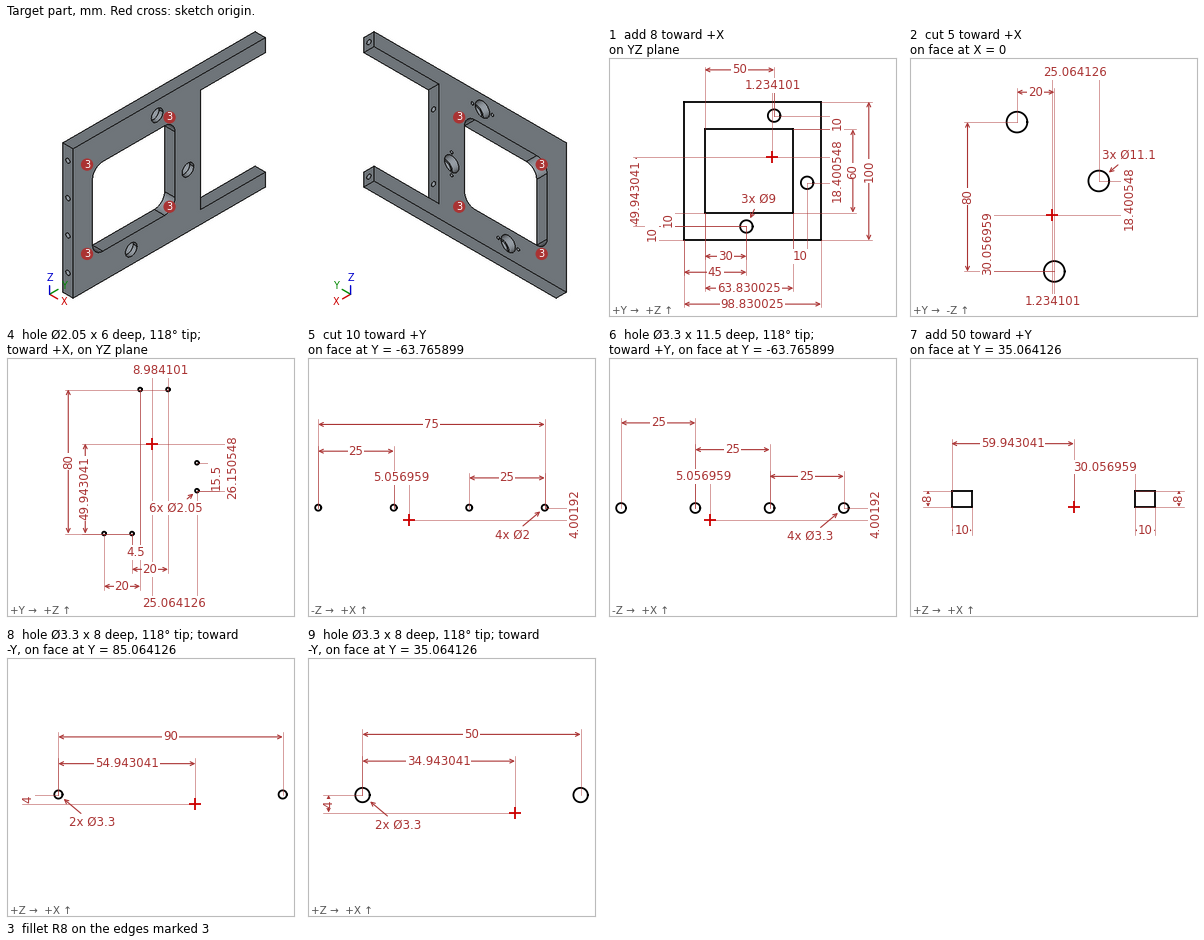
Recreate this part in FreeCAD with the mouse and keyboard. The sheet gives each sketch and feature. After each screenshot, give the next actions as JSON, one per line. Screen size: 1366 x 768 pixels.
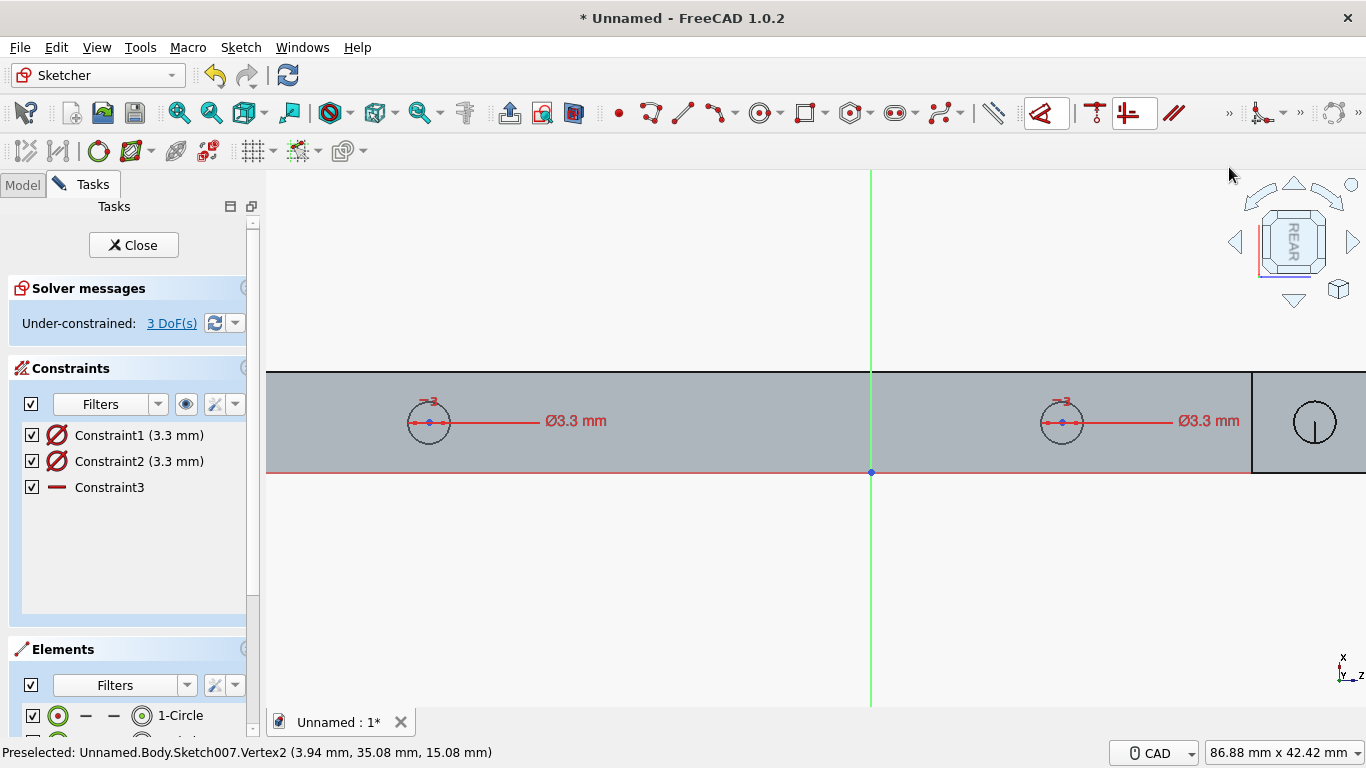
{"action": "left_click", "coordinate": [429, 423]}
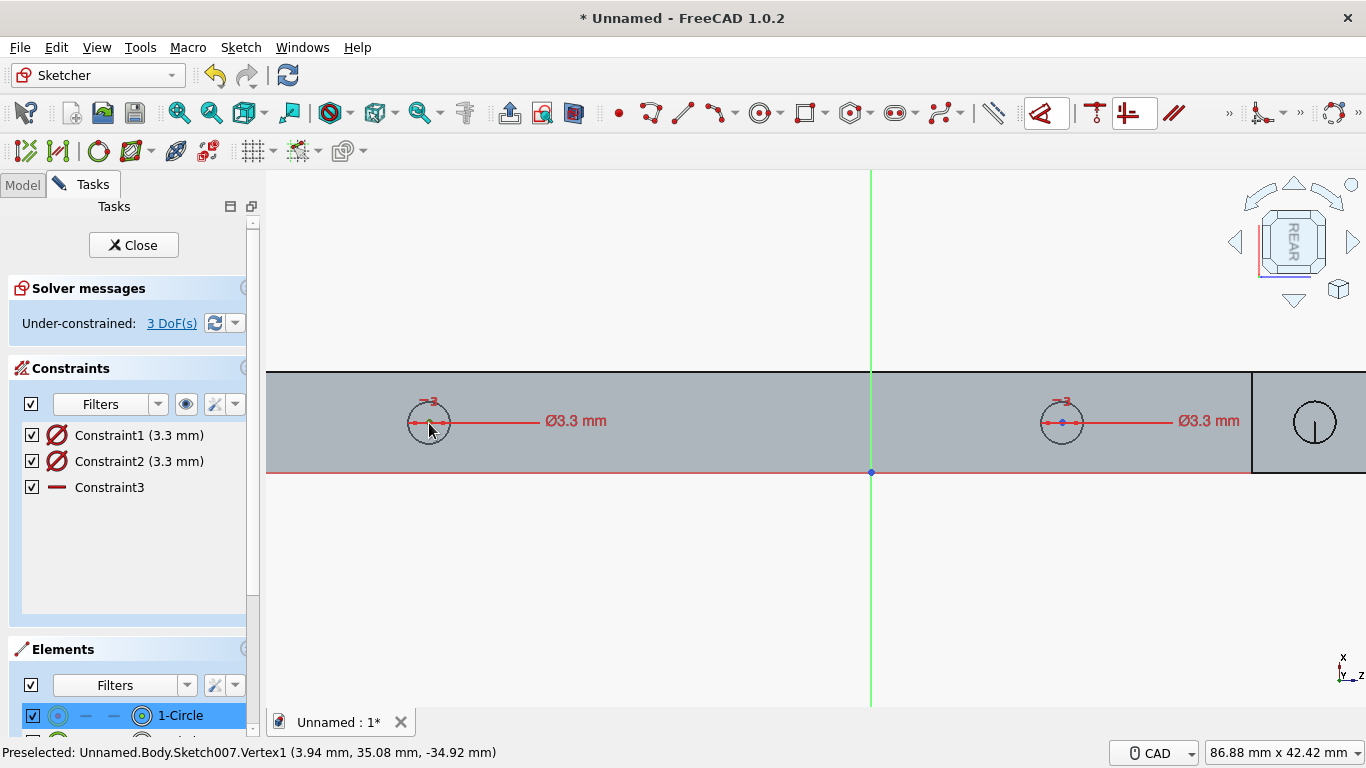
{"action": "key", "text": "i"}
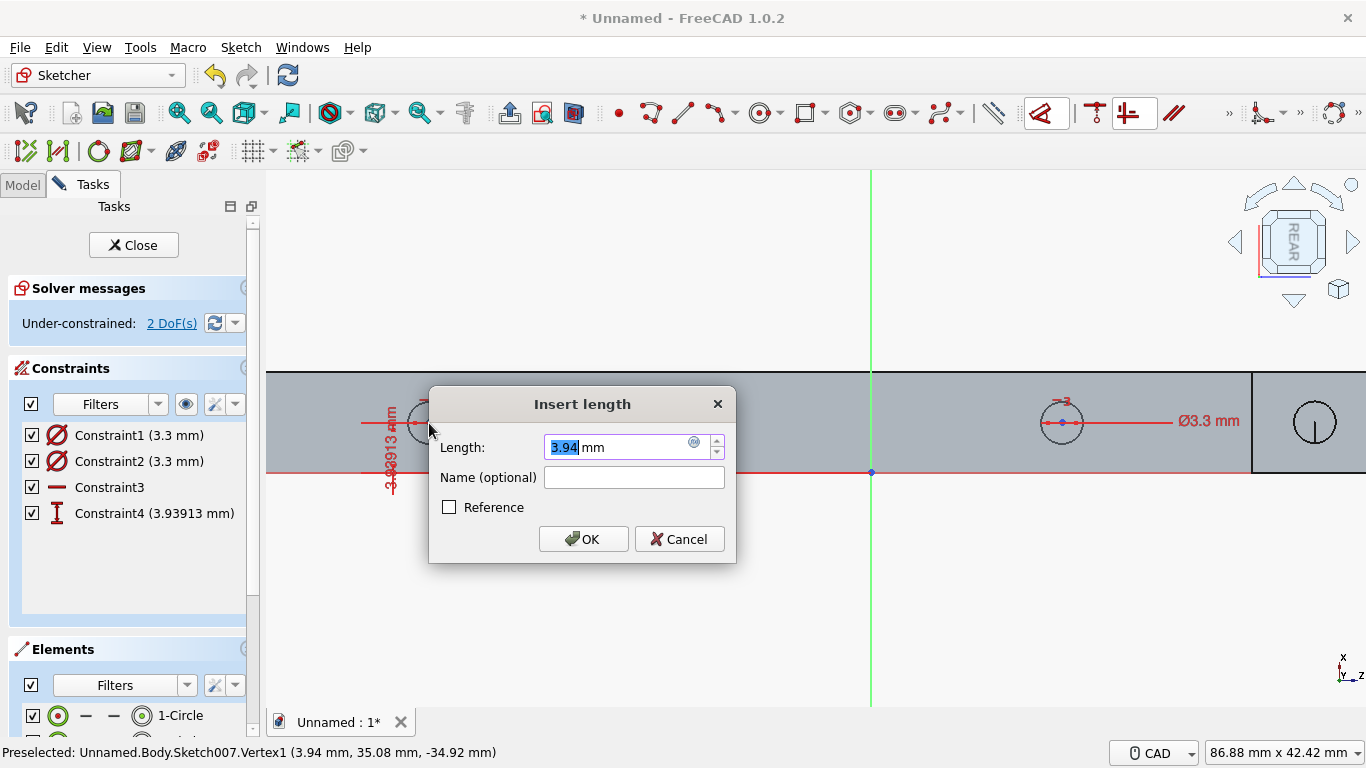
{"action": "type", "text": "4"}
{"action": "key", "text": "Return"}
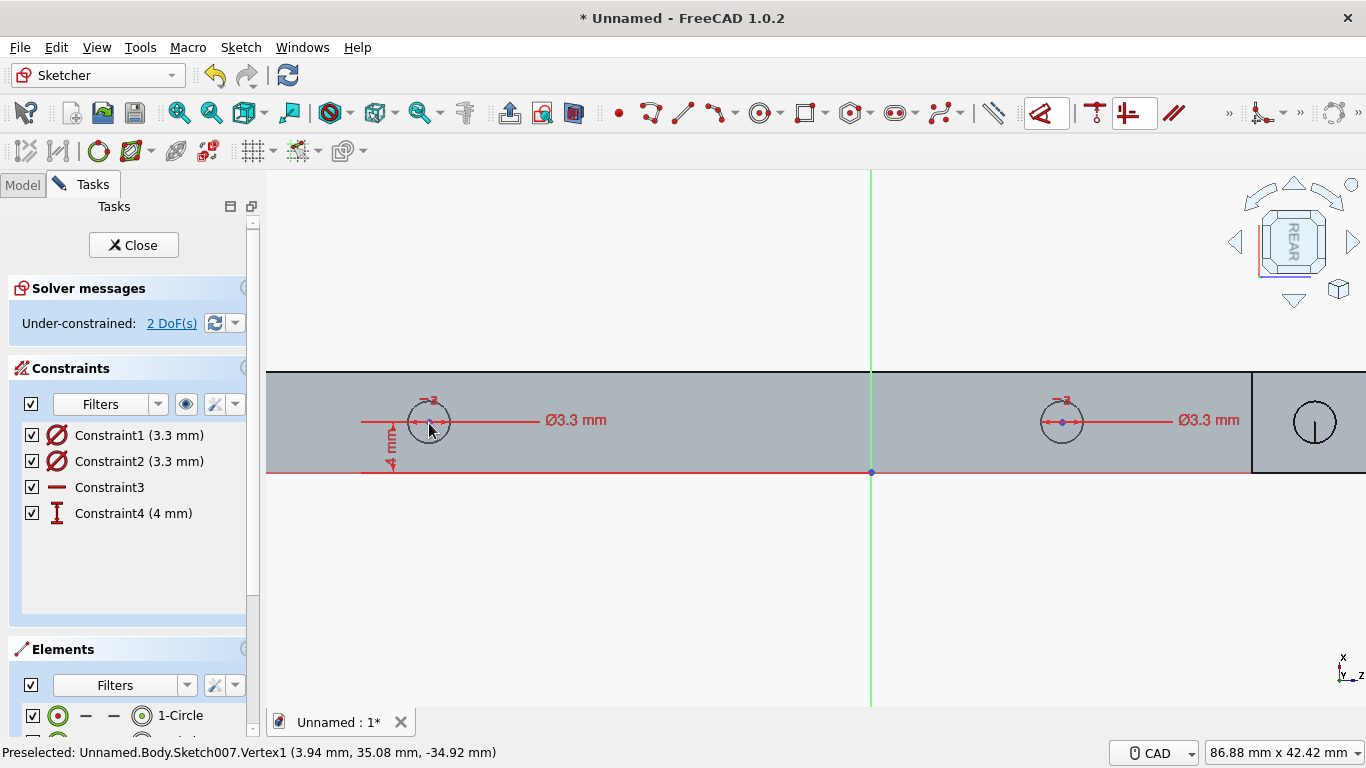
{"action": "left_click", "coordinate": [429, 422]}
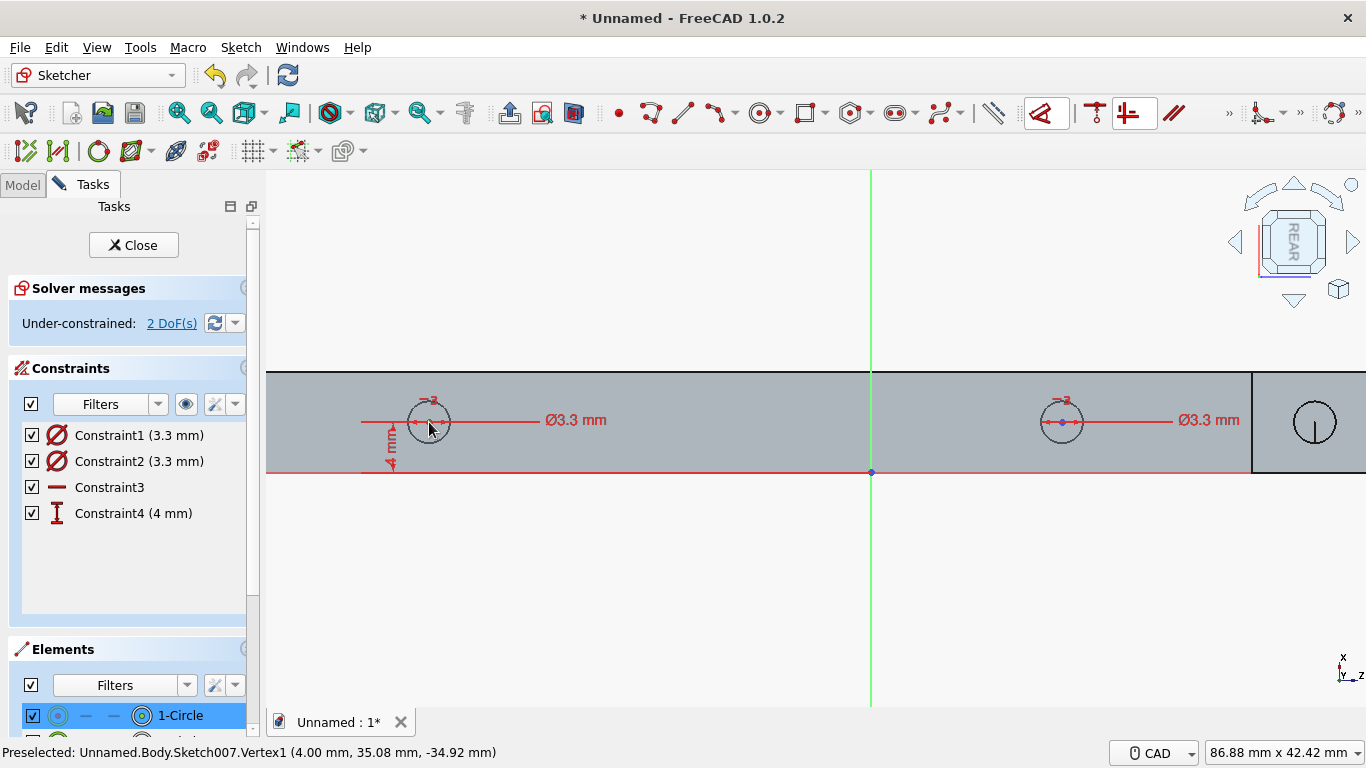
{"action": "left_click", "coordinate": [1062, 422]}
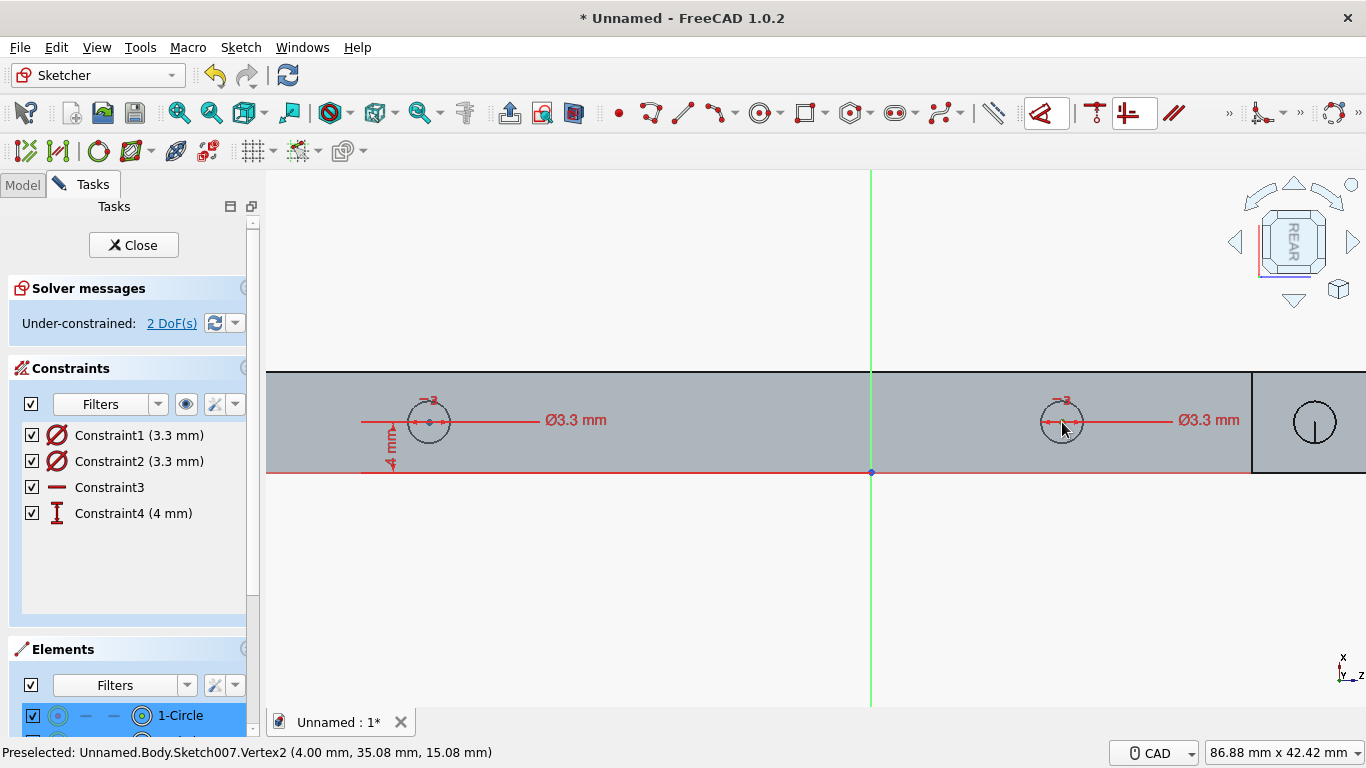
{"action": "key", "text": "l"}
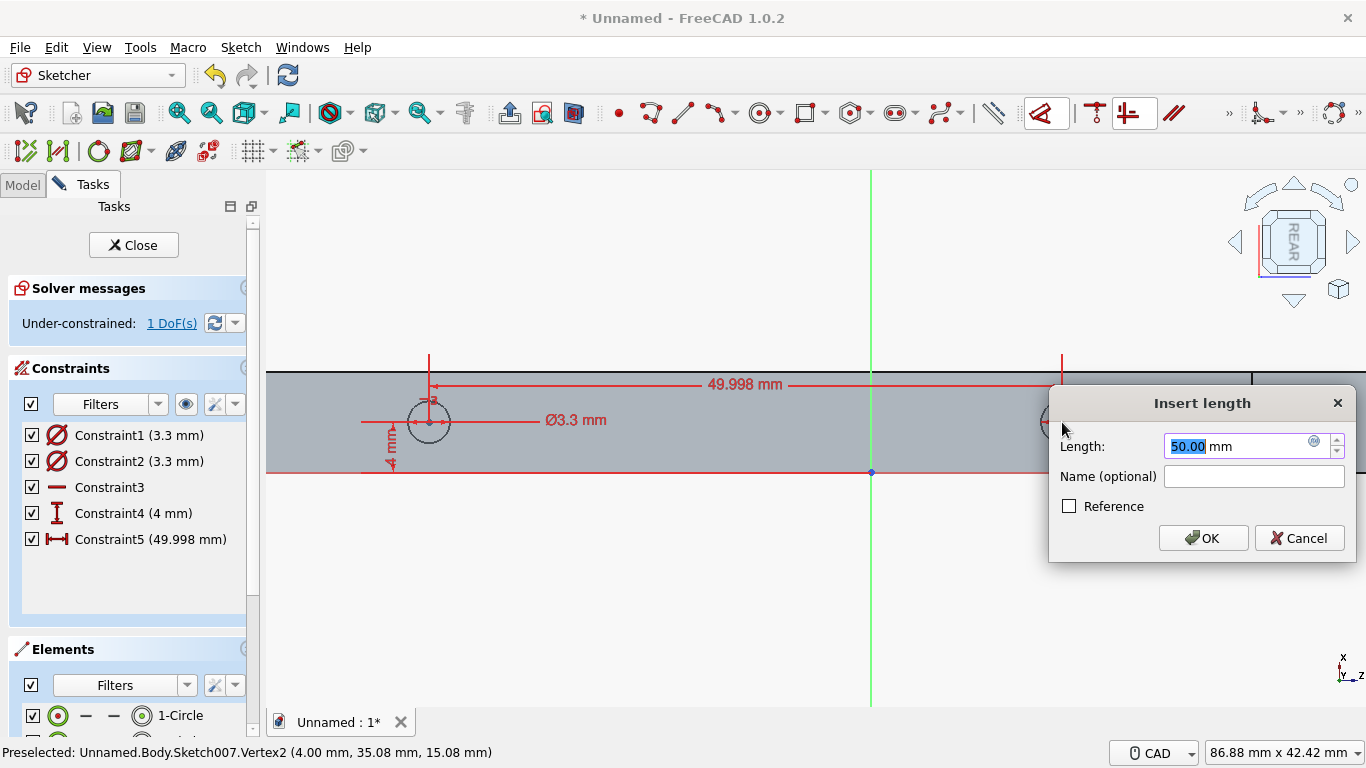
{"action": "type", "text": "50"}
{"action": "key", "text": "Return"}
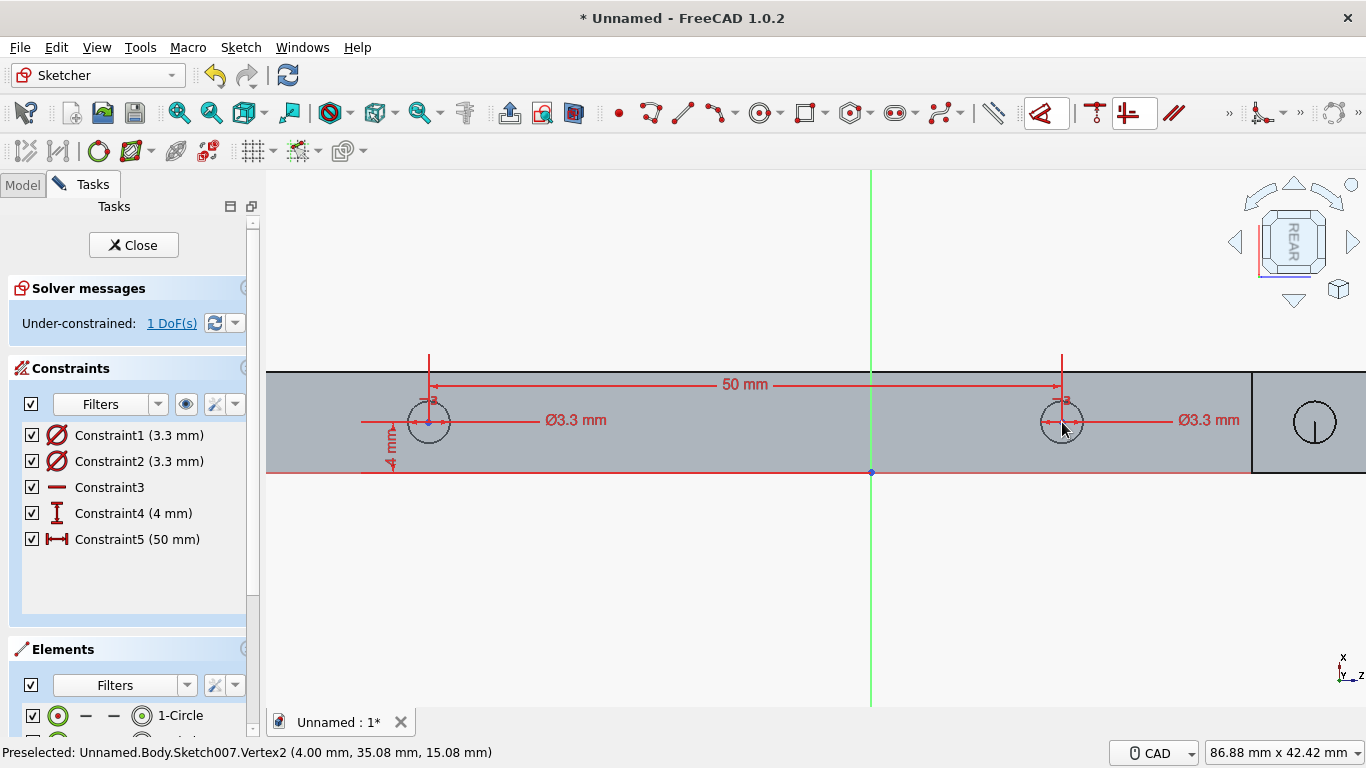
{"action": "left_click", "coordinate": [429, 422]}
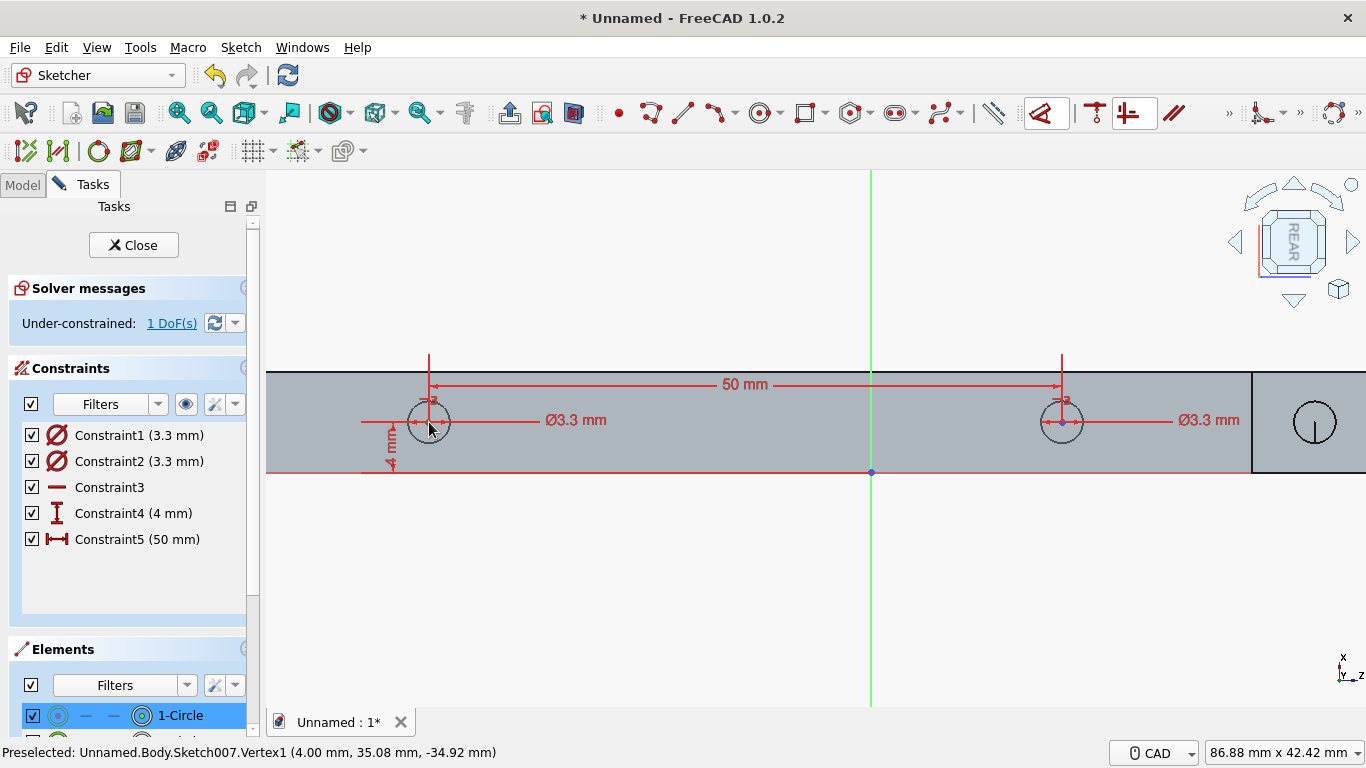
{"action": "key", "text": "l"}